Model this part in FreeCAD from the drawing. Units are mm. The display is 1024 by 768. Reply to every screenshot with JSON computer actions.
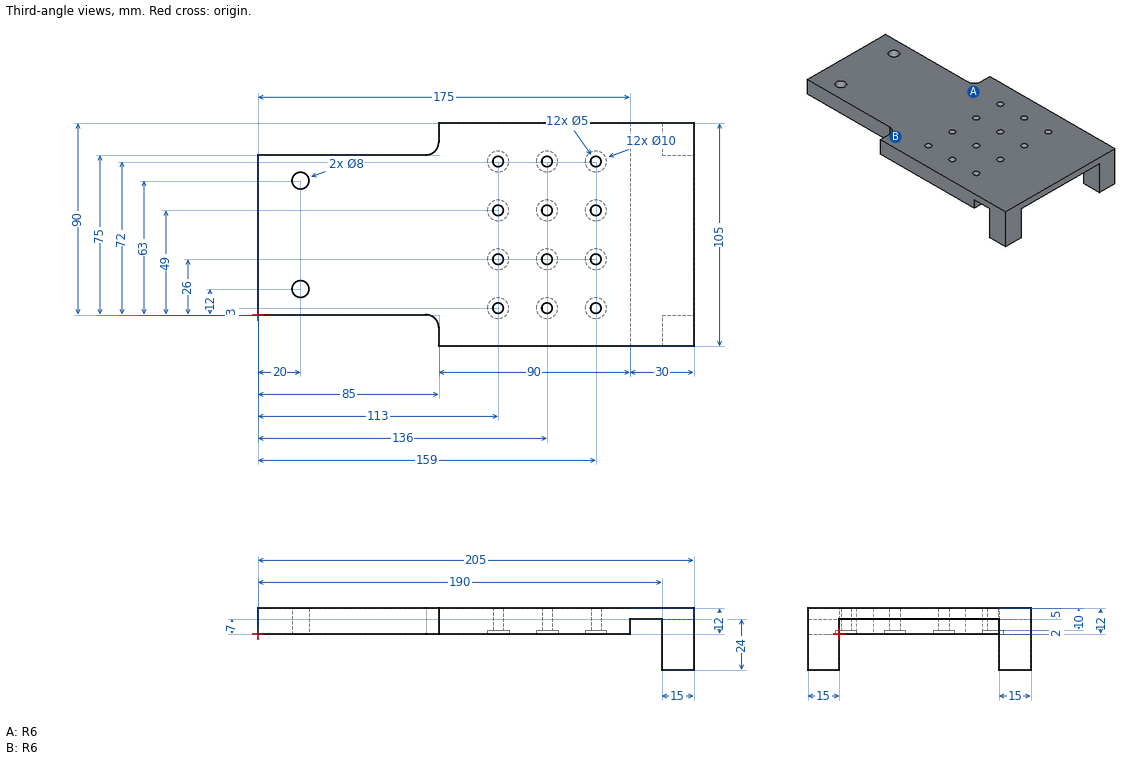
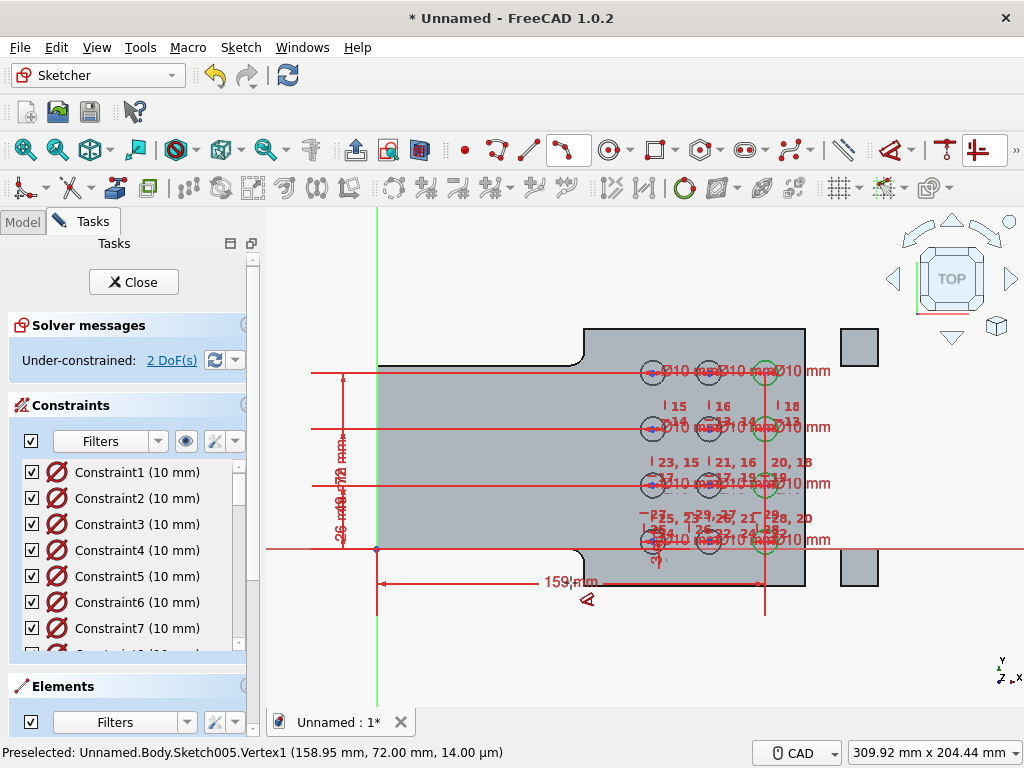
{"action": "left_click", "coordinate": [709, 373]}
{"action": "left_click", "coordinate": [466, 583]}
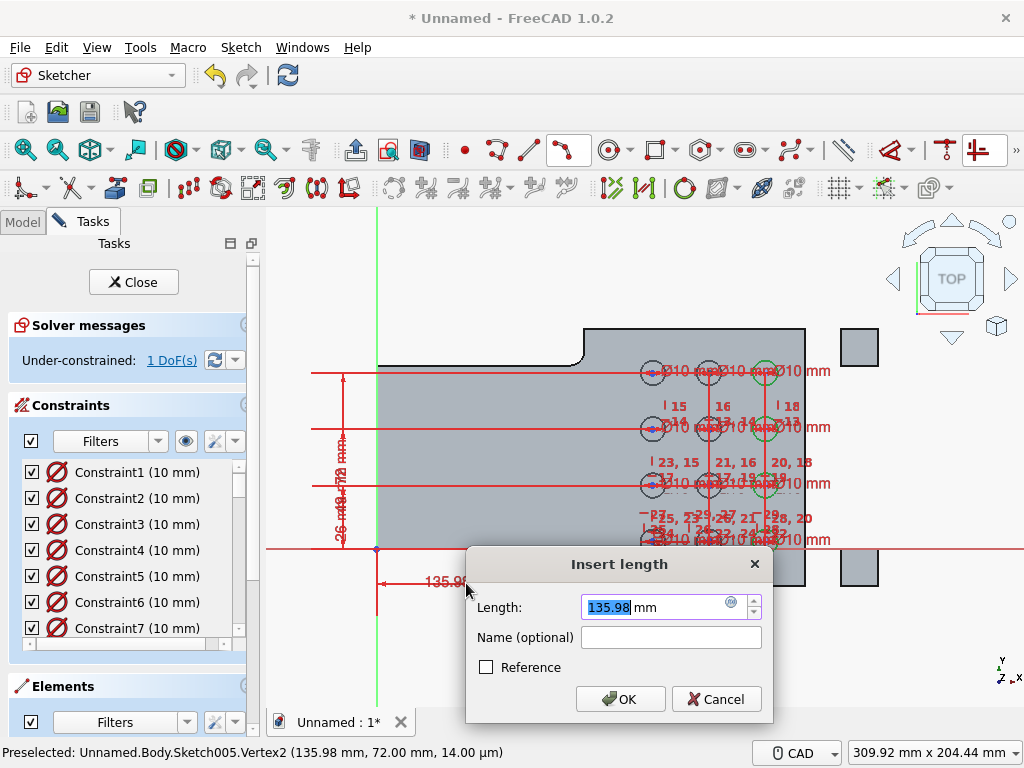
{"action": "type", "text": "136"}
{"action": "key", "text": "Return"}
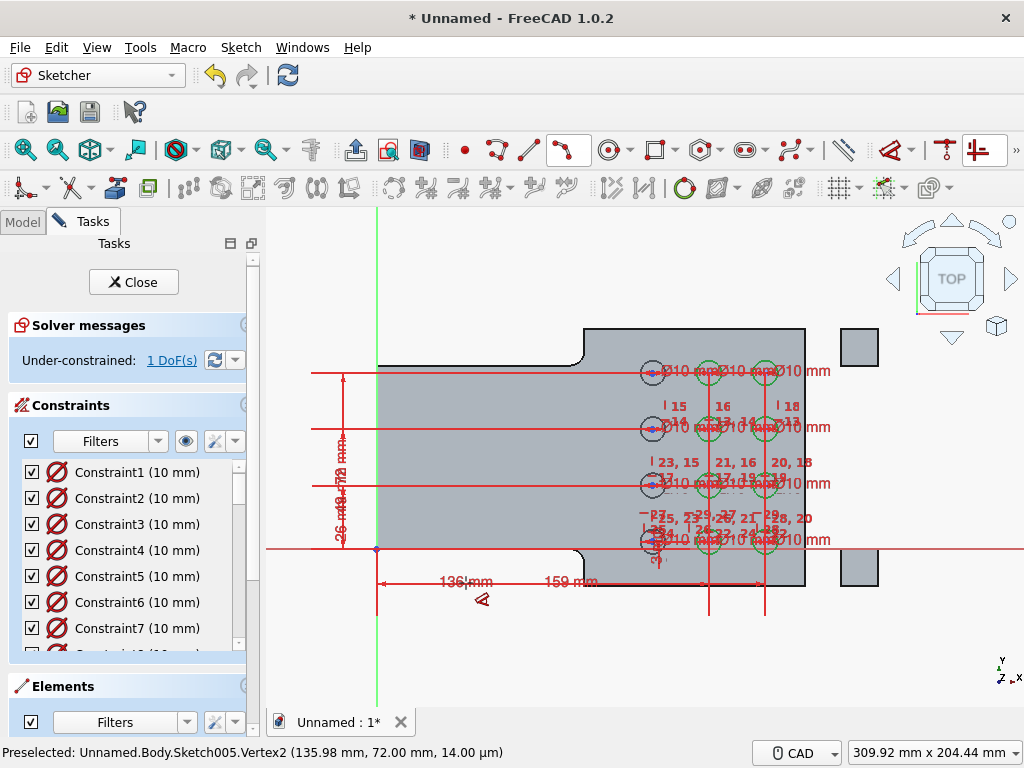
{"action": "left_click", "coordinate": [653, 373]}
{"action": "left_click", "coordinate": [515, 339]}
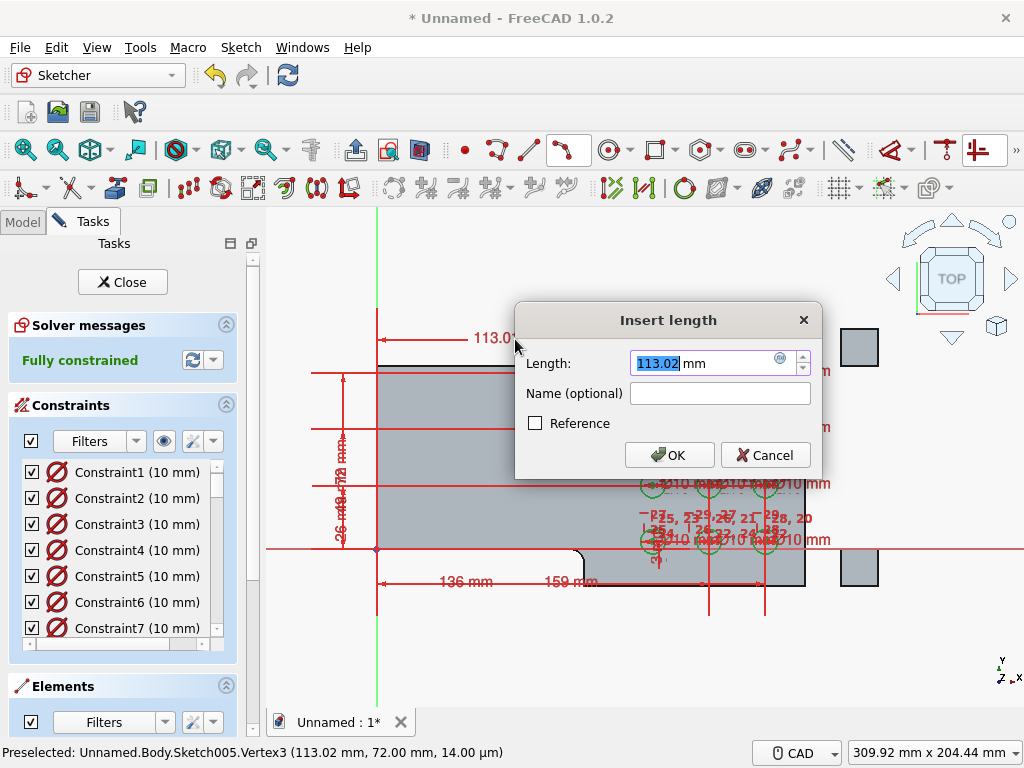
{"action": "type", "text": "113"}
{"action": "key", "text": "Return"}
{"action": "key", "text": "Escape"}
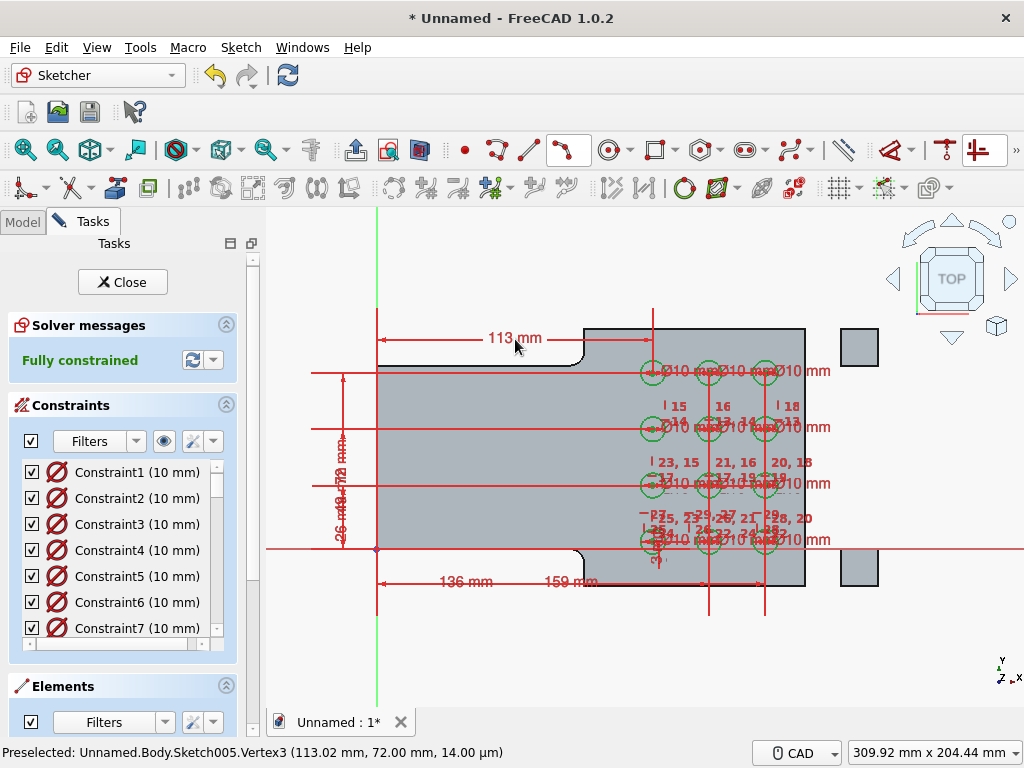
{"action": "left_click", "coordinate": [123, 282]}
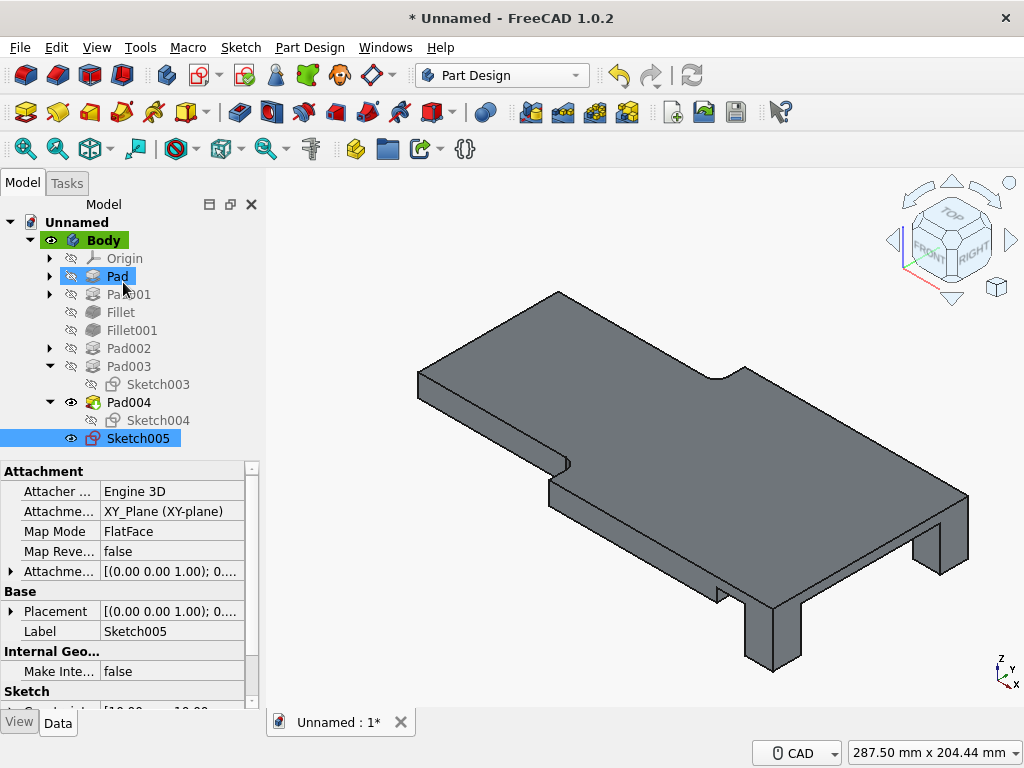
{"action": "left_click", "coordinate": [240, 112]}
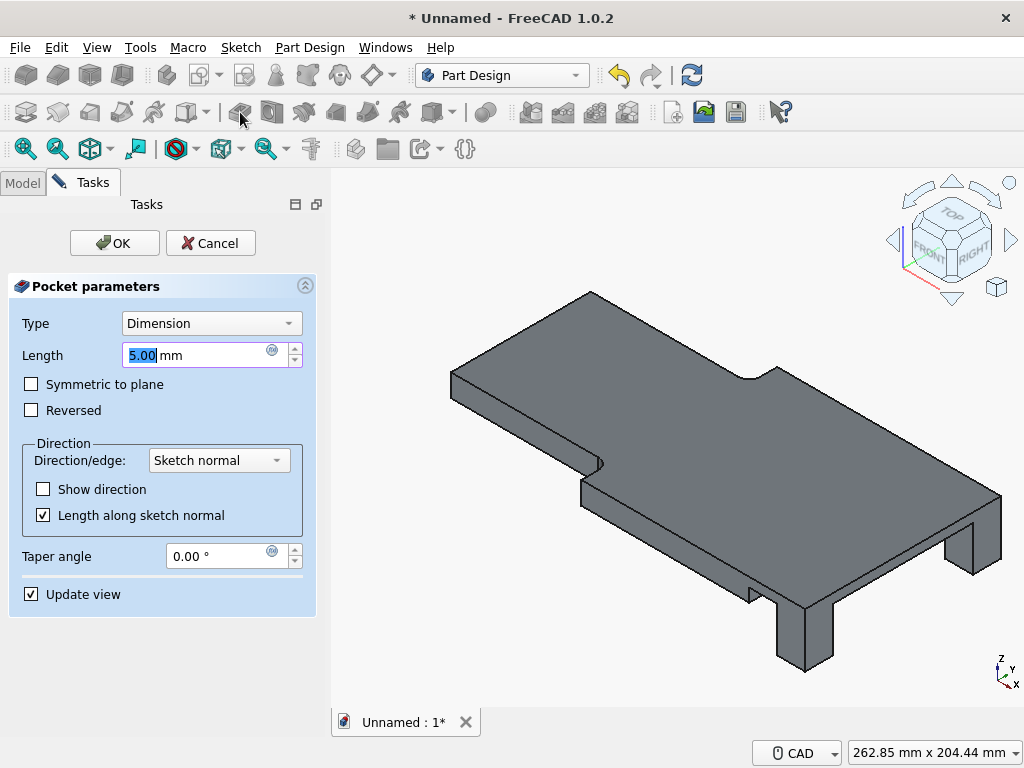
{"action": "type", "text": "2"}
{"action": "key", "text": "Tab"}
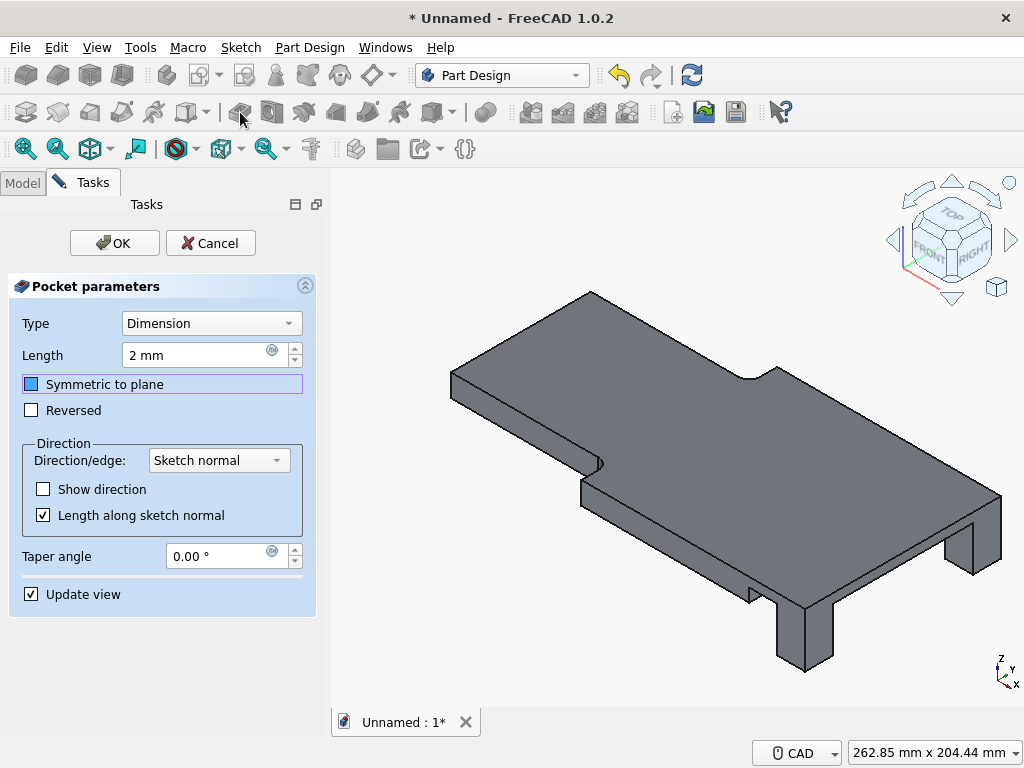
{"action": "left_click", "coordinate": [30, 410]}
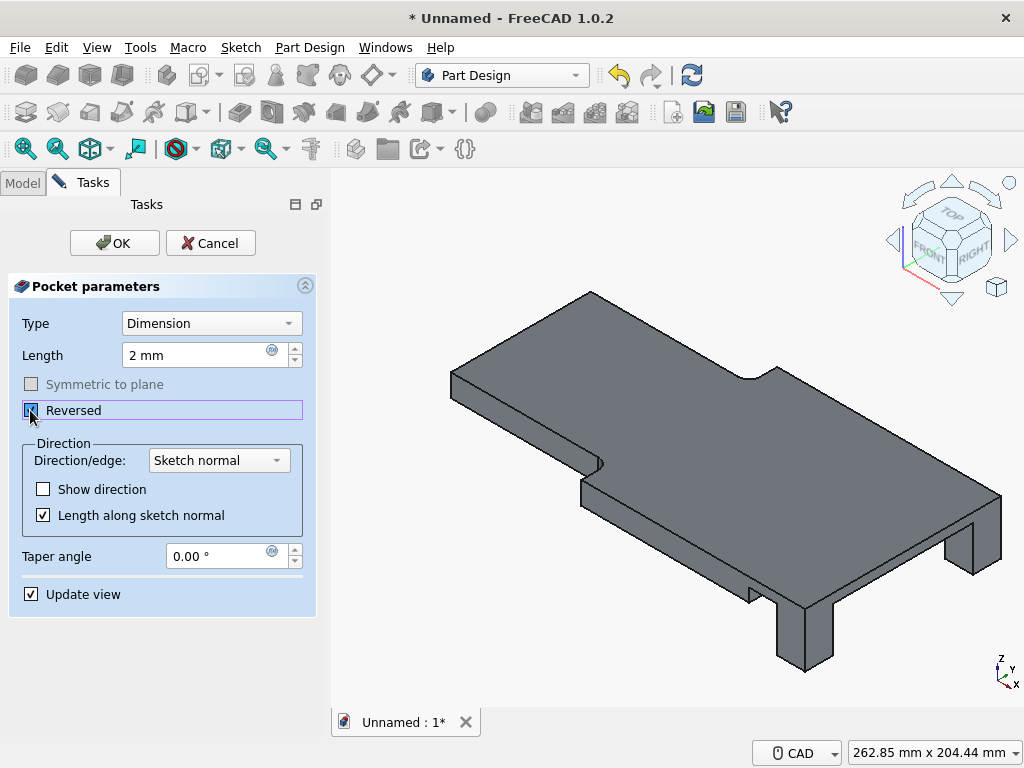
{"action": "left_click", "coordinate": [115, 243]}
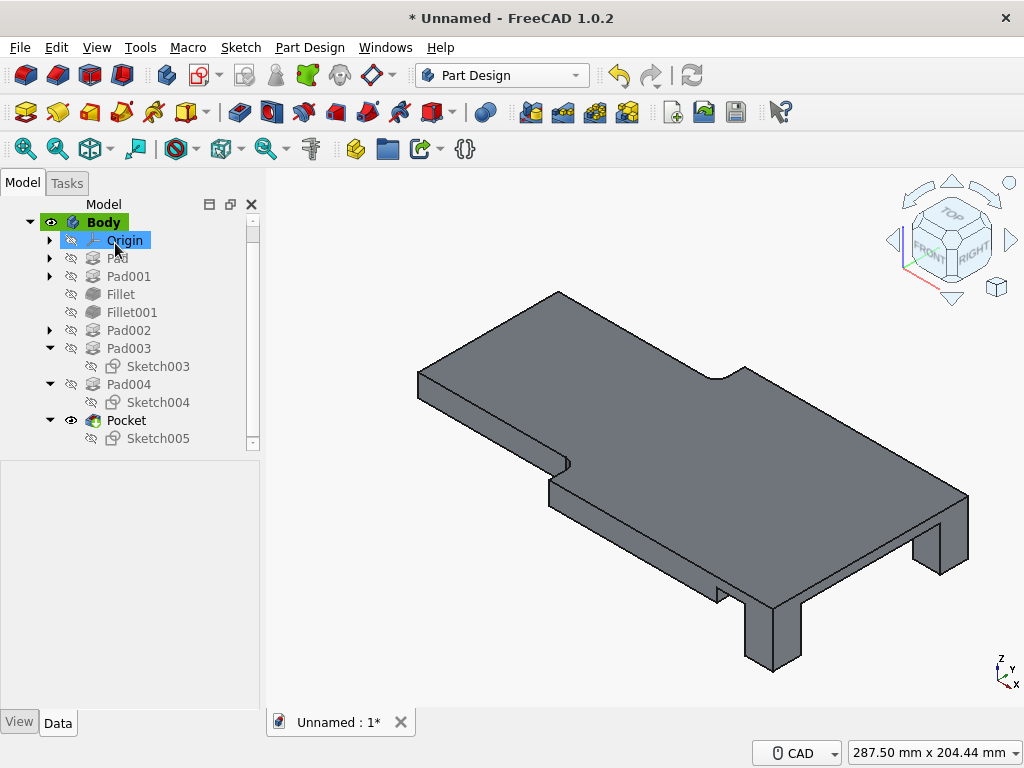
{"action": "key", "text": "5"}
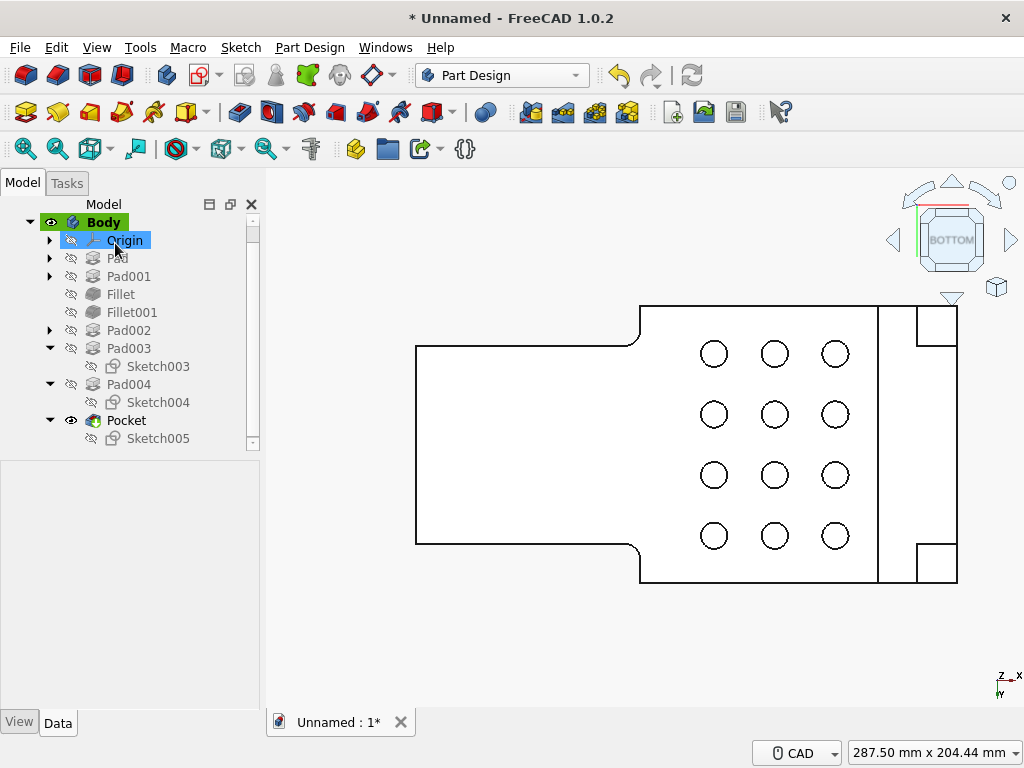
{"action": "left_click", "coordinate": [714, 535]}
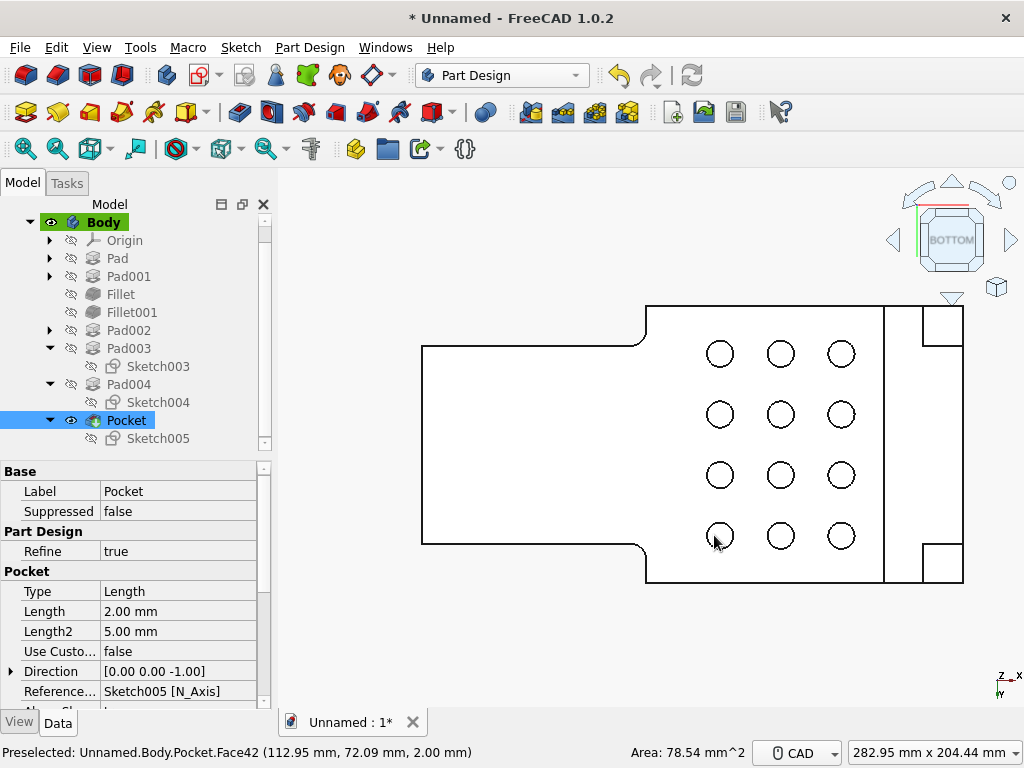
{"action": "left_click", "coordinate": [200, 76]}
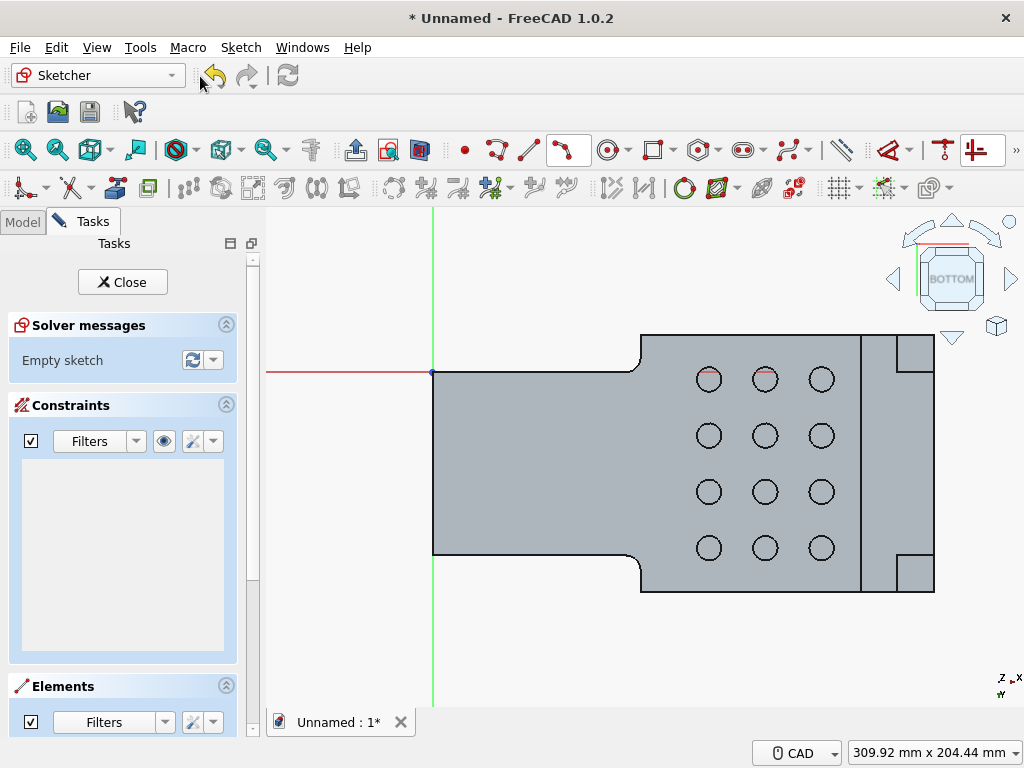
{"action": "left_click", "coordinate": [608, 150]}